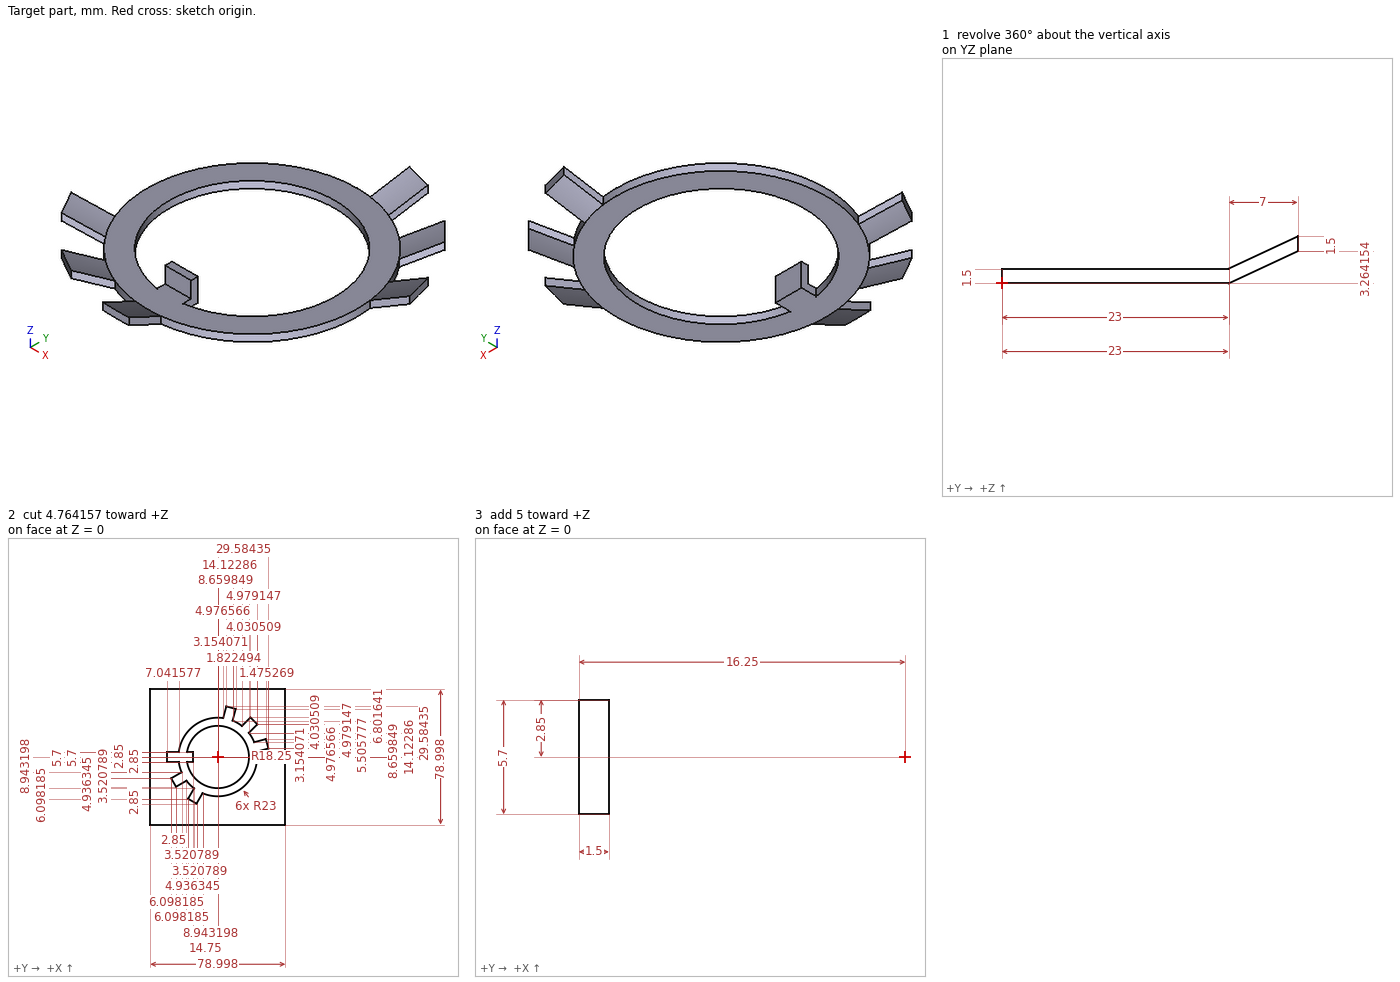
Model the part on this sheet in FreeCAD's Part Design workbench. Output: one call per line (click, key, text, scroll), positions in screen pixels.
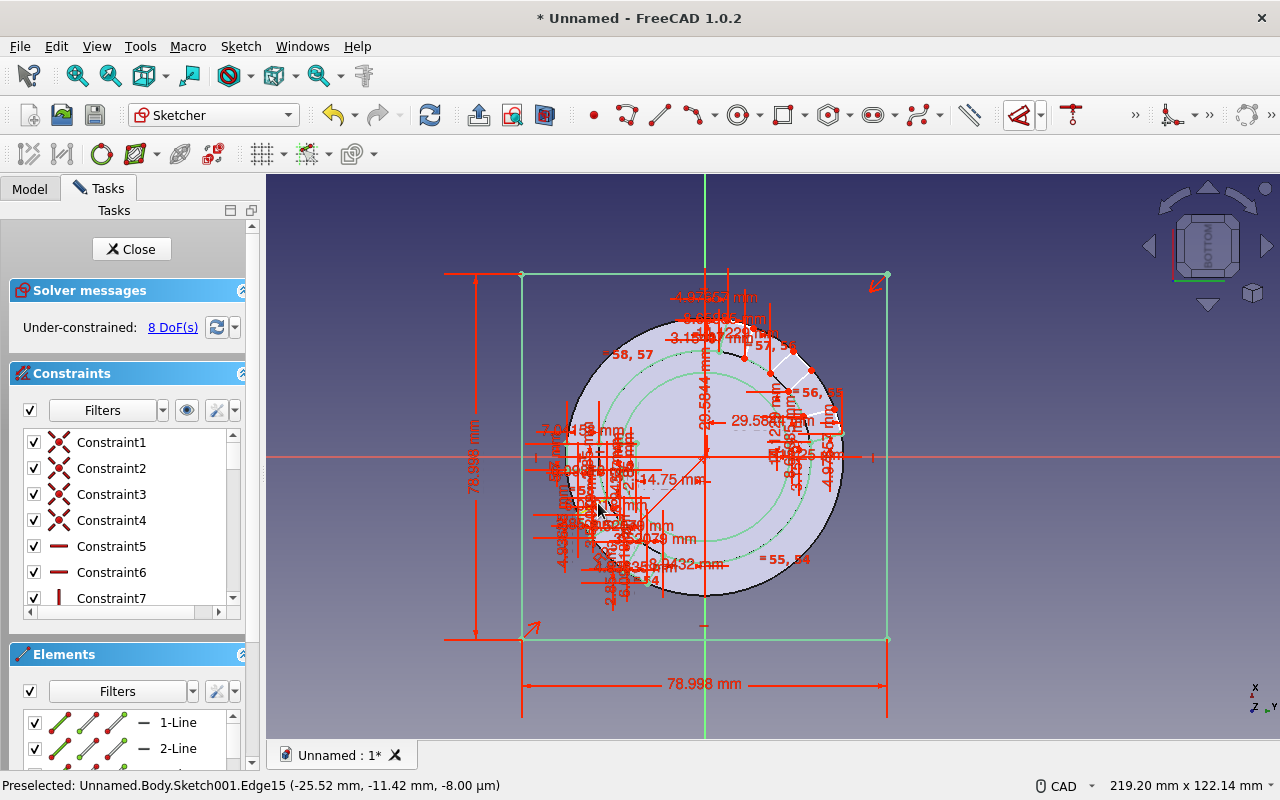
scroll(839, 427, up, 9)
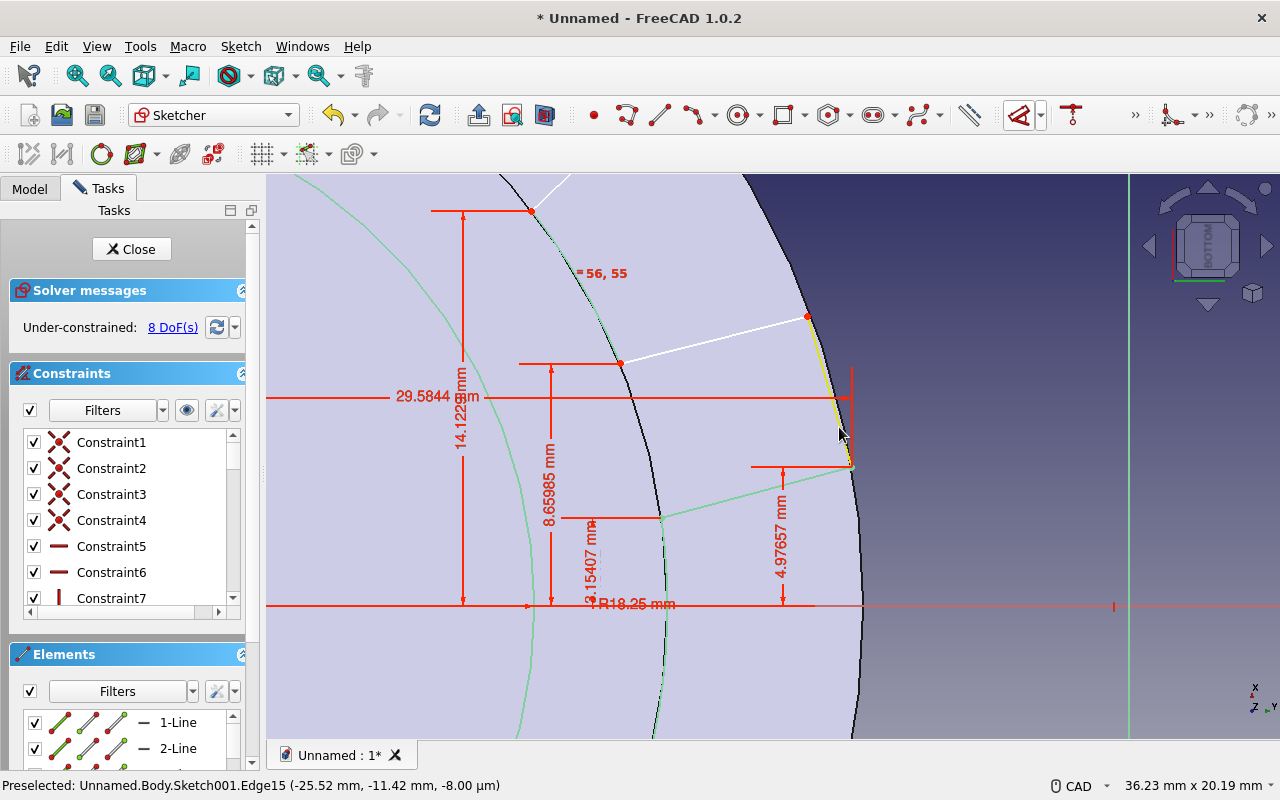
click(838, 422)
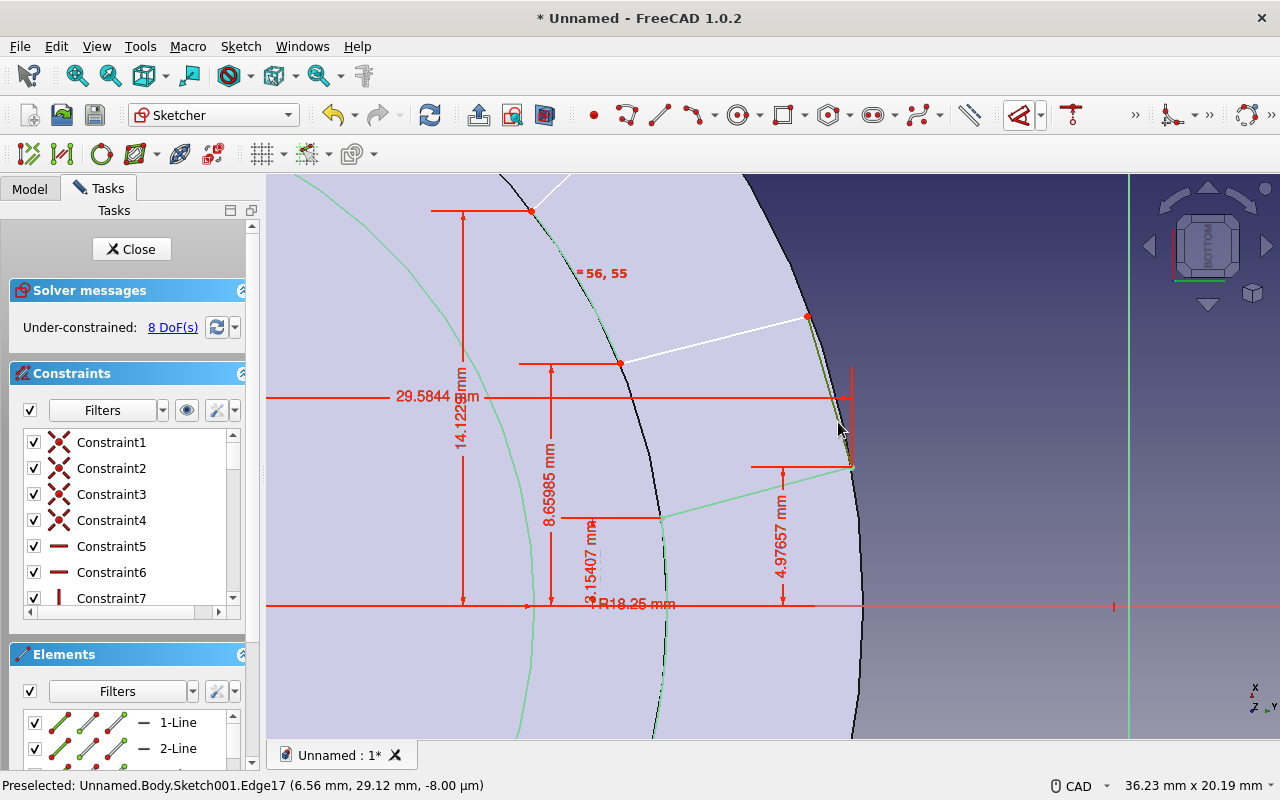
key(l)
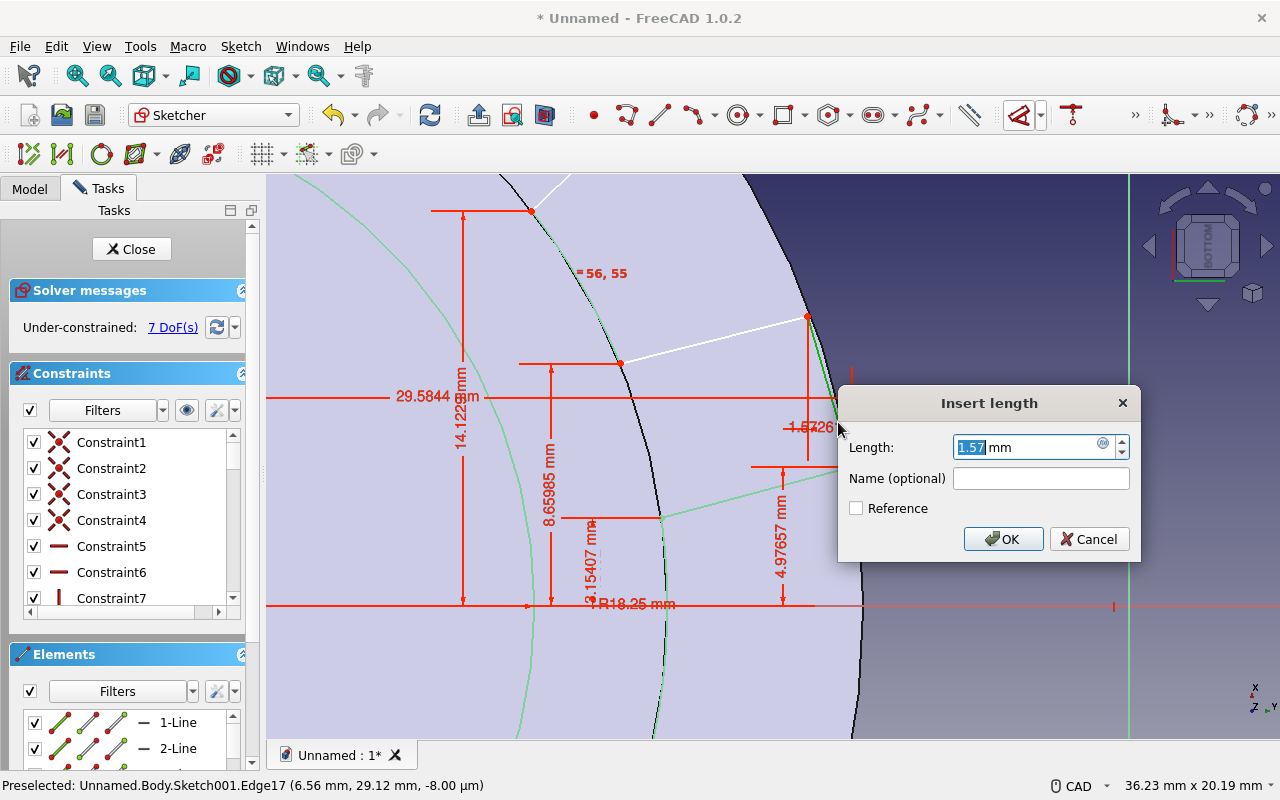
text(1.475269)
key(Return)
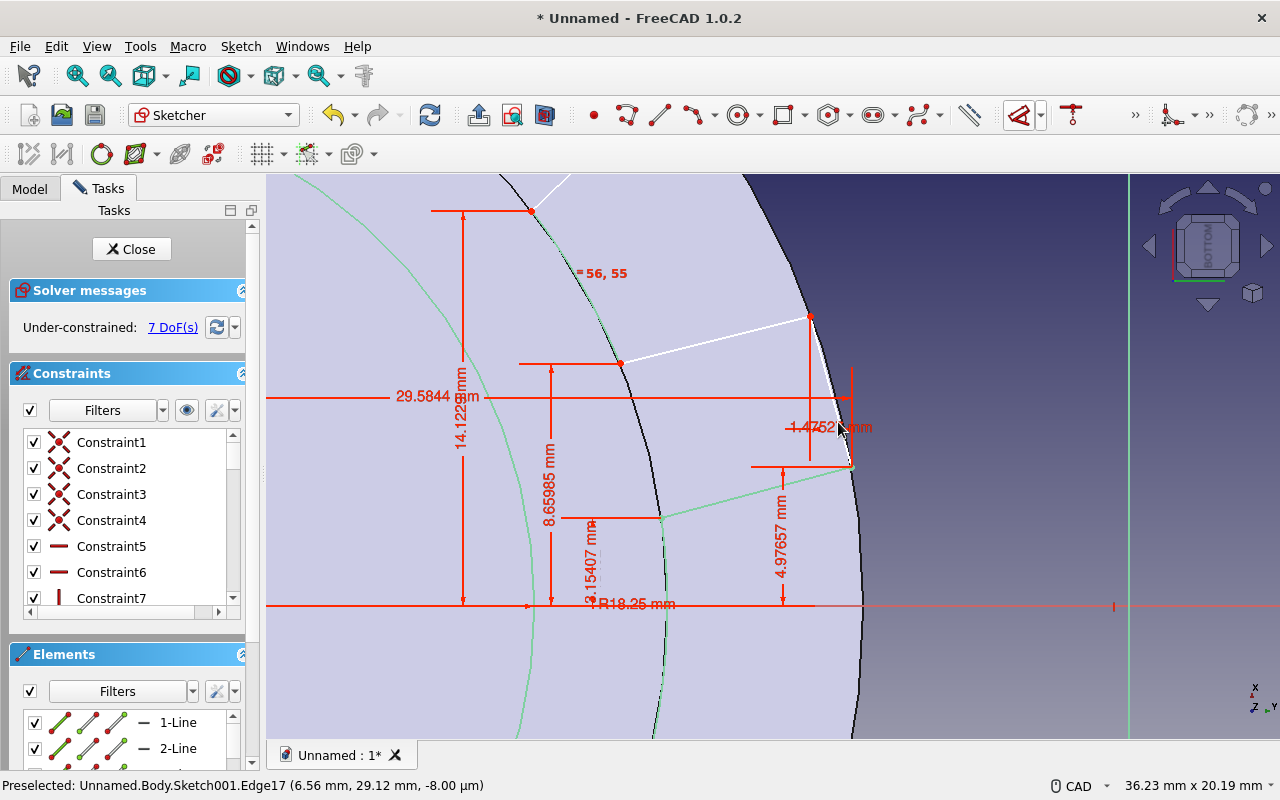
scroll(839, 427, down, 9)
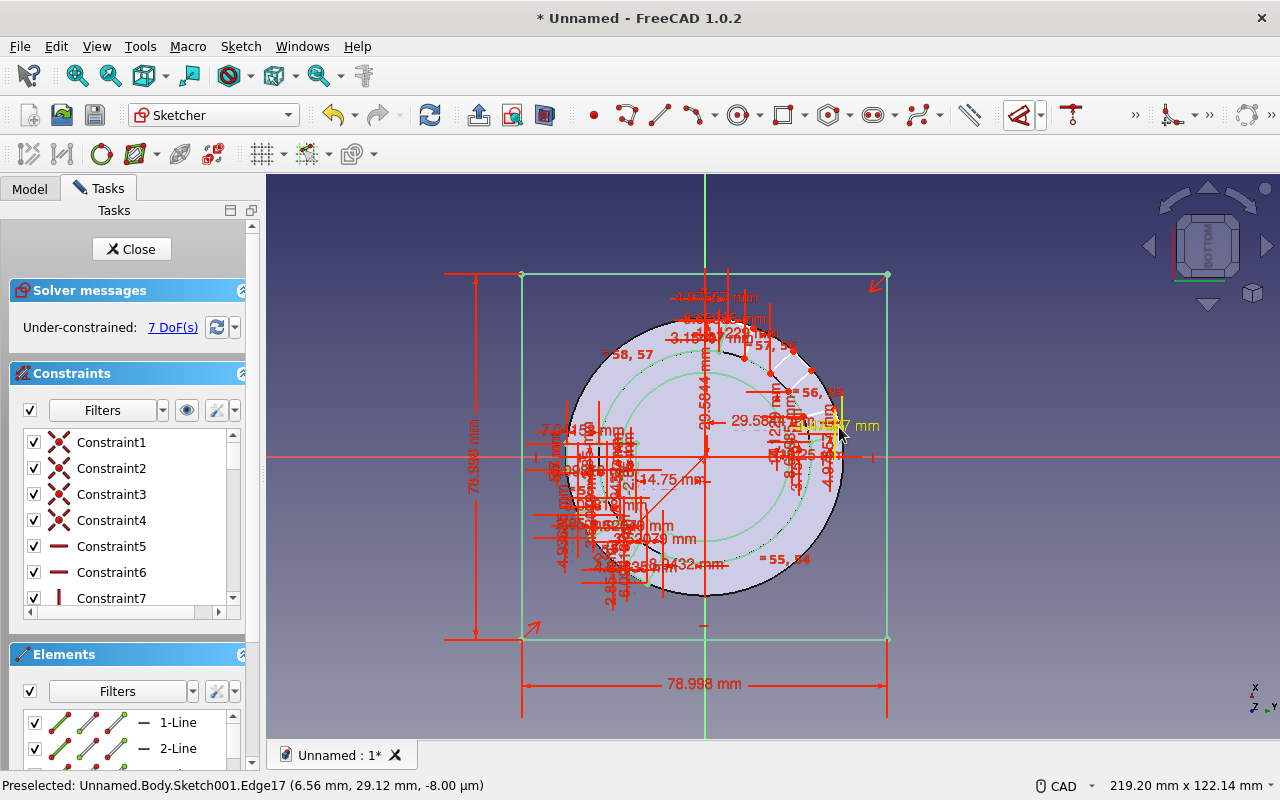
scroll(840, 427, up, 3)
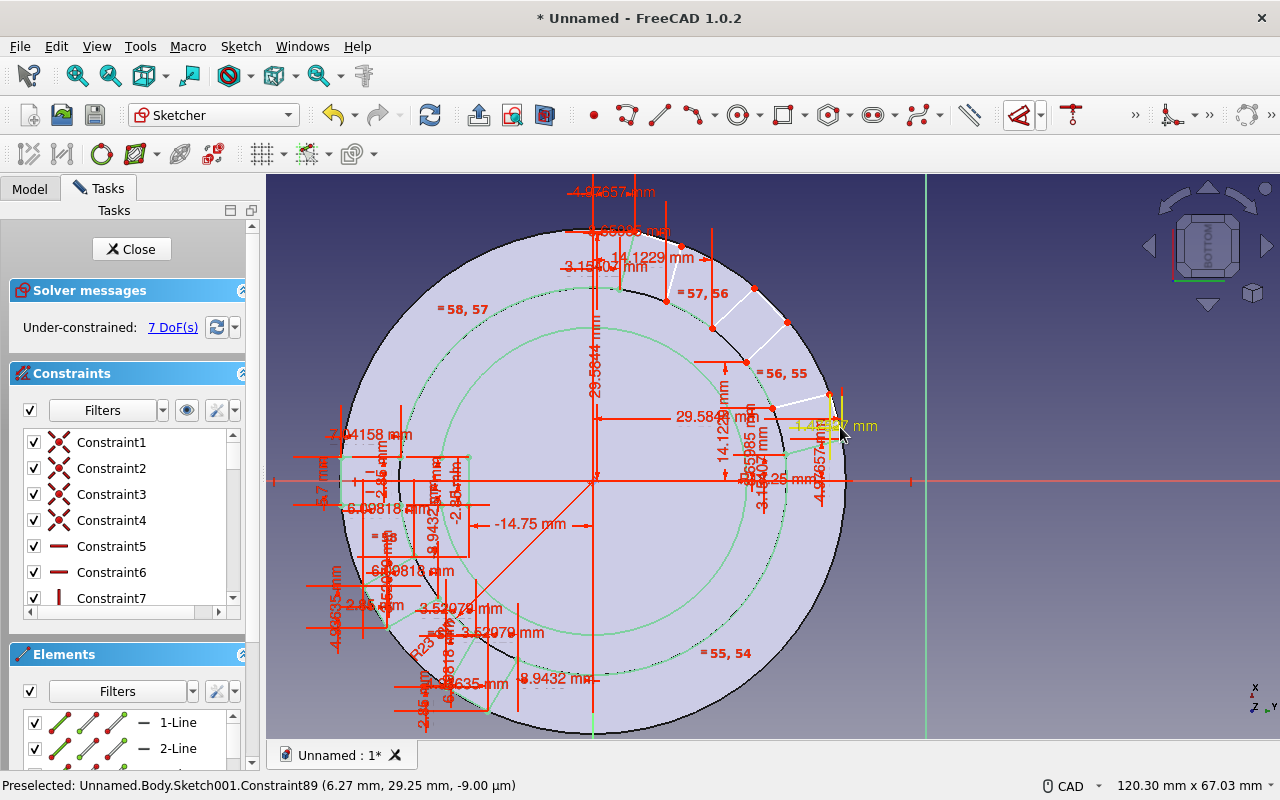
click(834, 408)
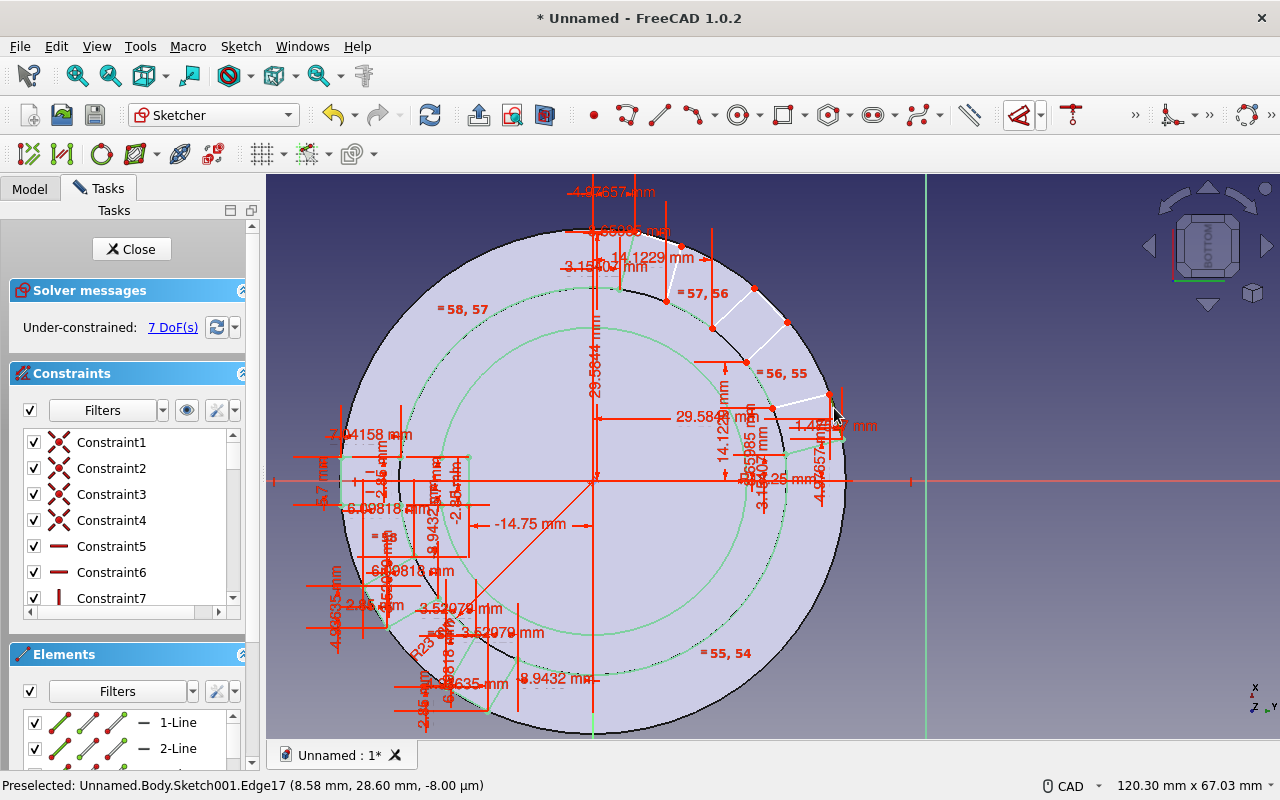
key(i)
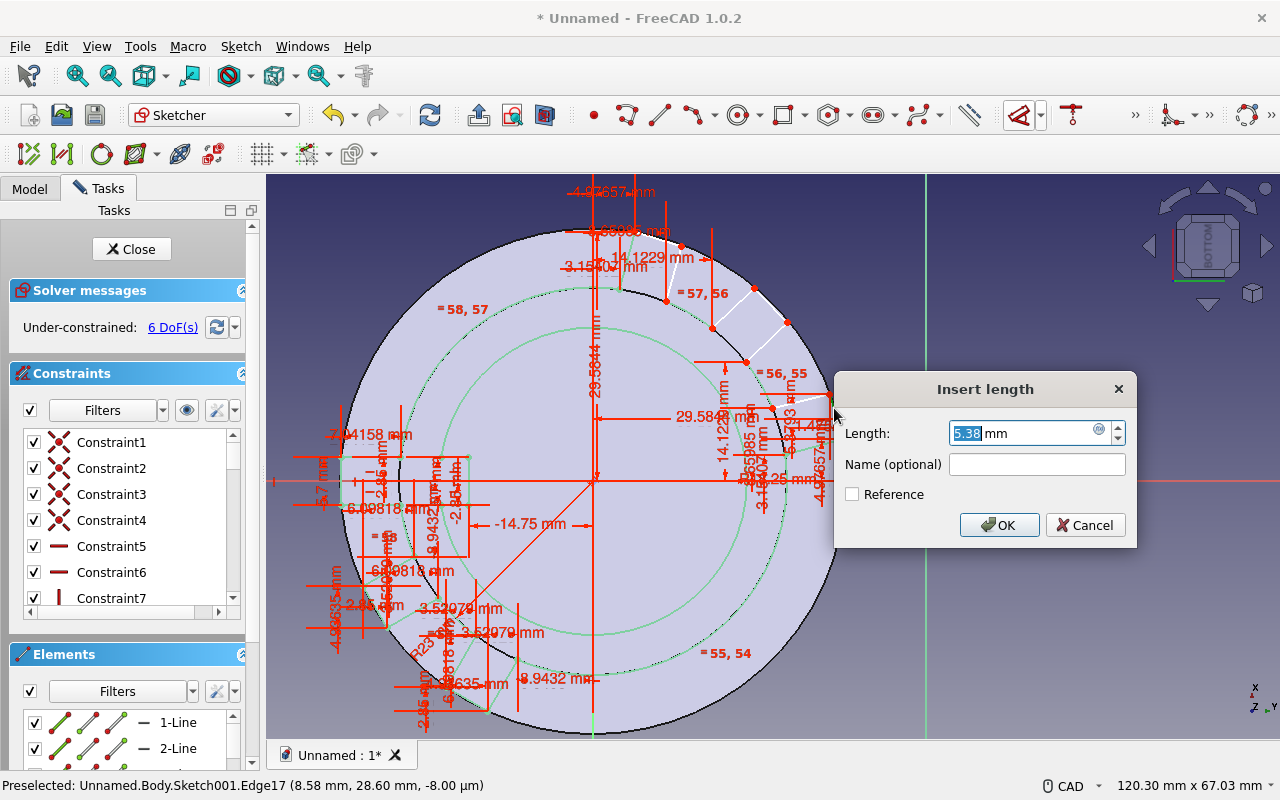
text(5.505777)
key(Return)